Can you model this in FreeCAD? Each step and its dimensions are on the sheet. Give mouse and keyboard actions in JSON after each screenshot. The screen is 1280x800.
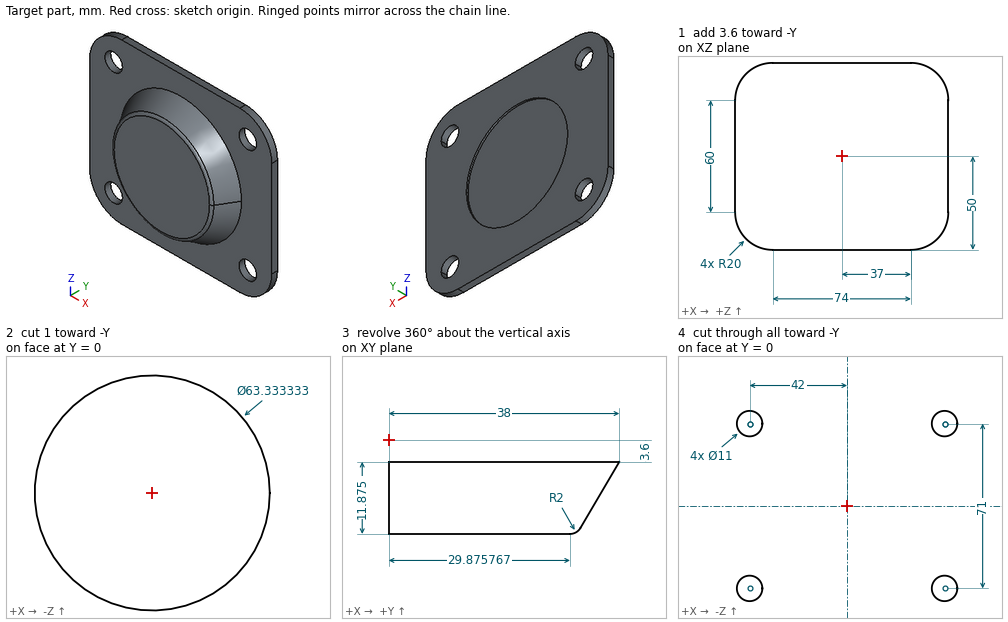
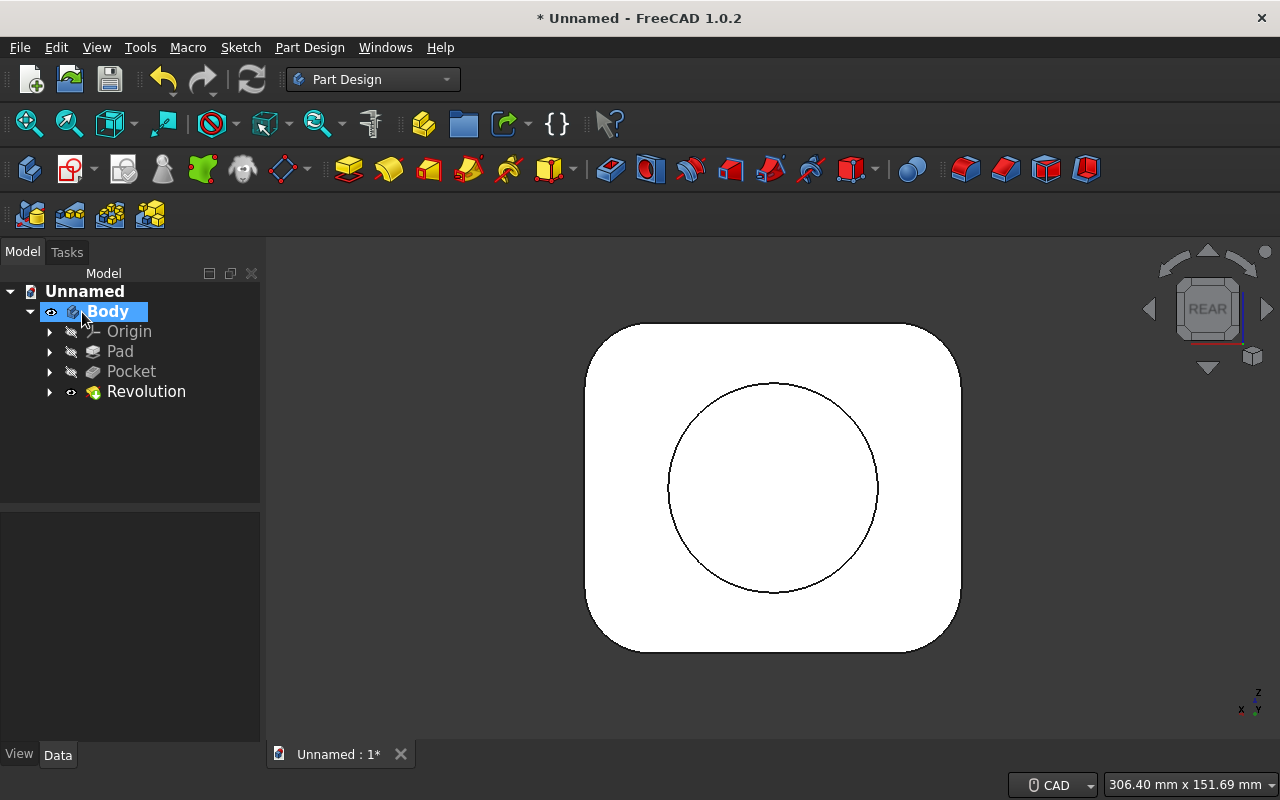
{"action": "left_click", "coordinate": [665, 582]}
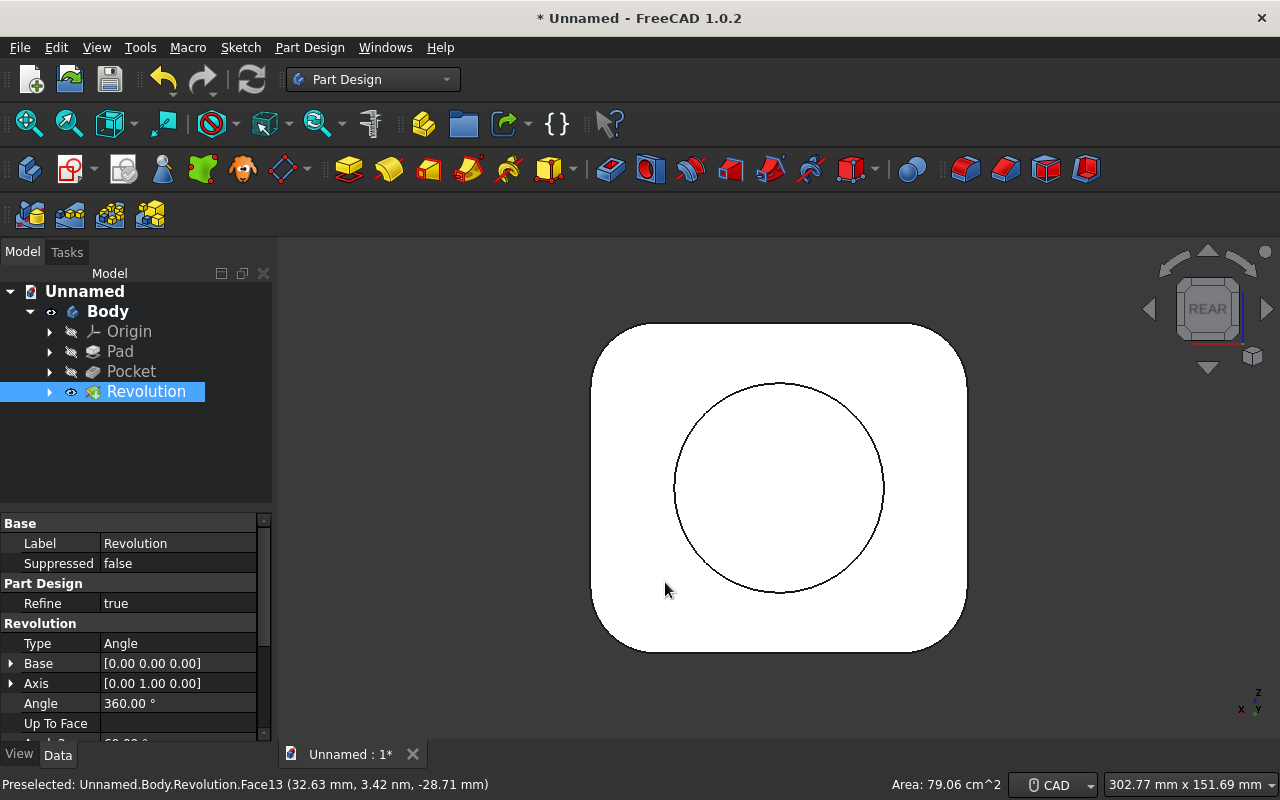
{"action": "left_click", "coordinate": [70, 170]}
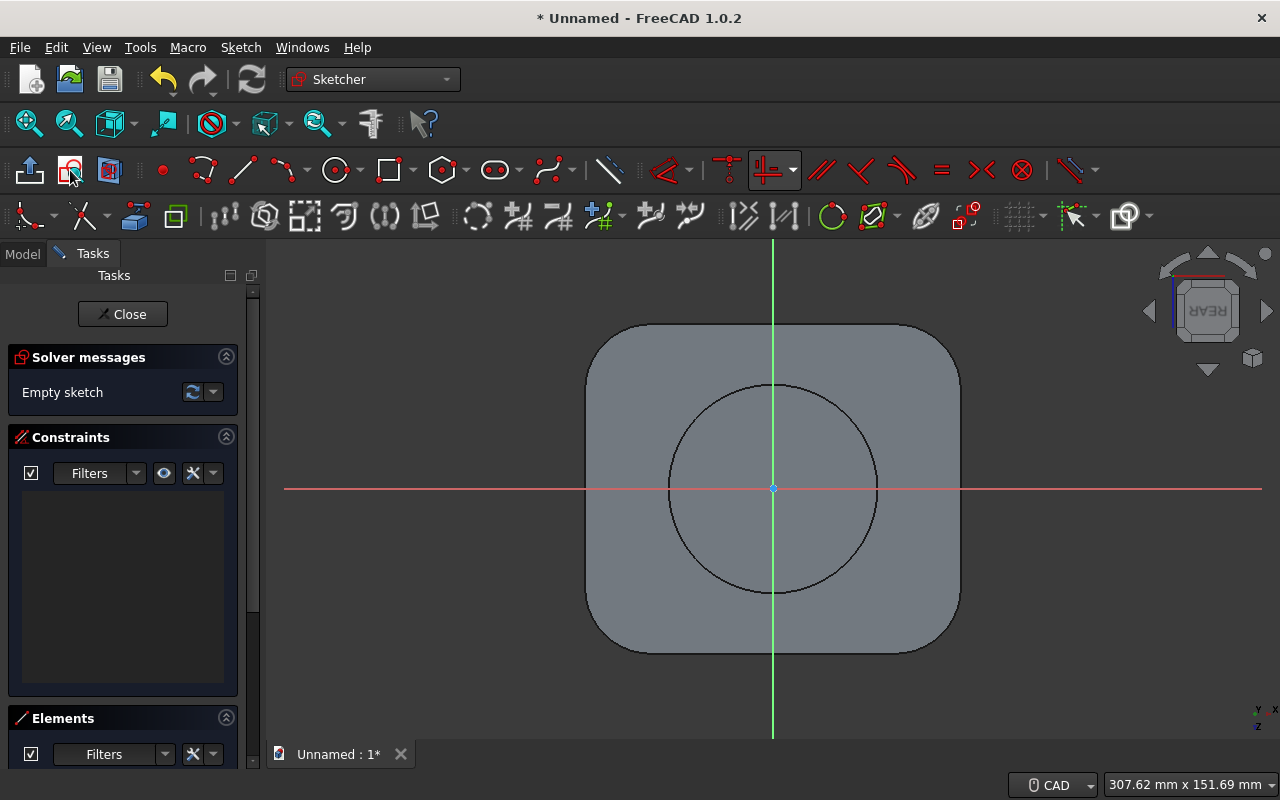
{"action": "left_click", "coordinate": [336, 170]}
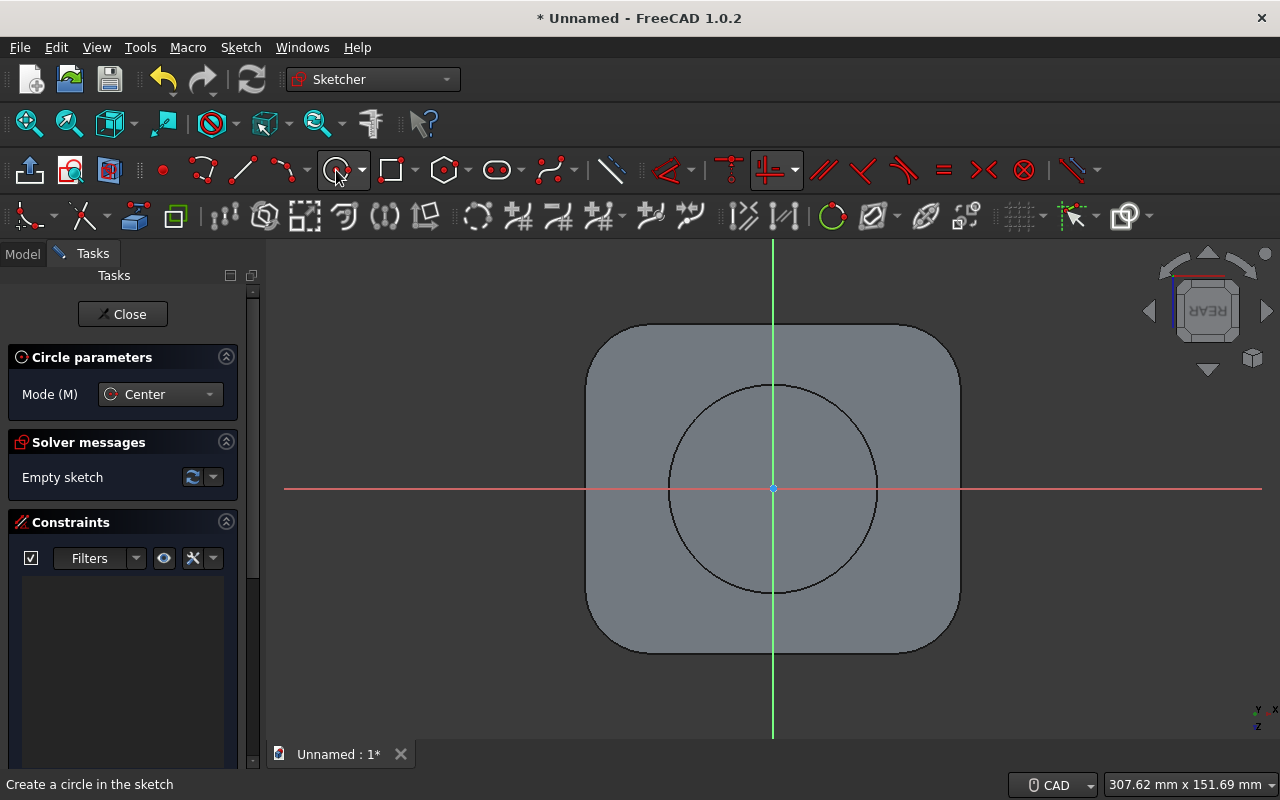
{"action": "scroll", "coordinate": [635, 372], "scroll_direction": "up", "scroll_amount": 2}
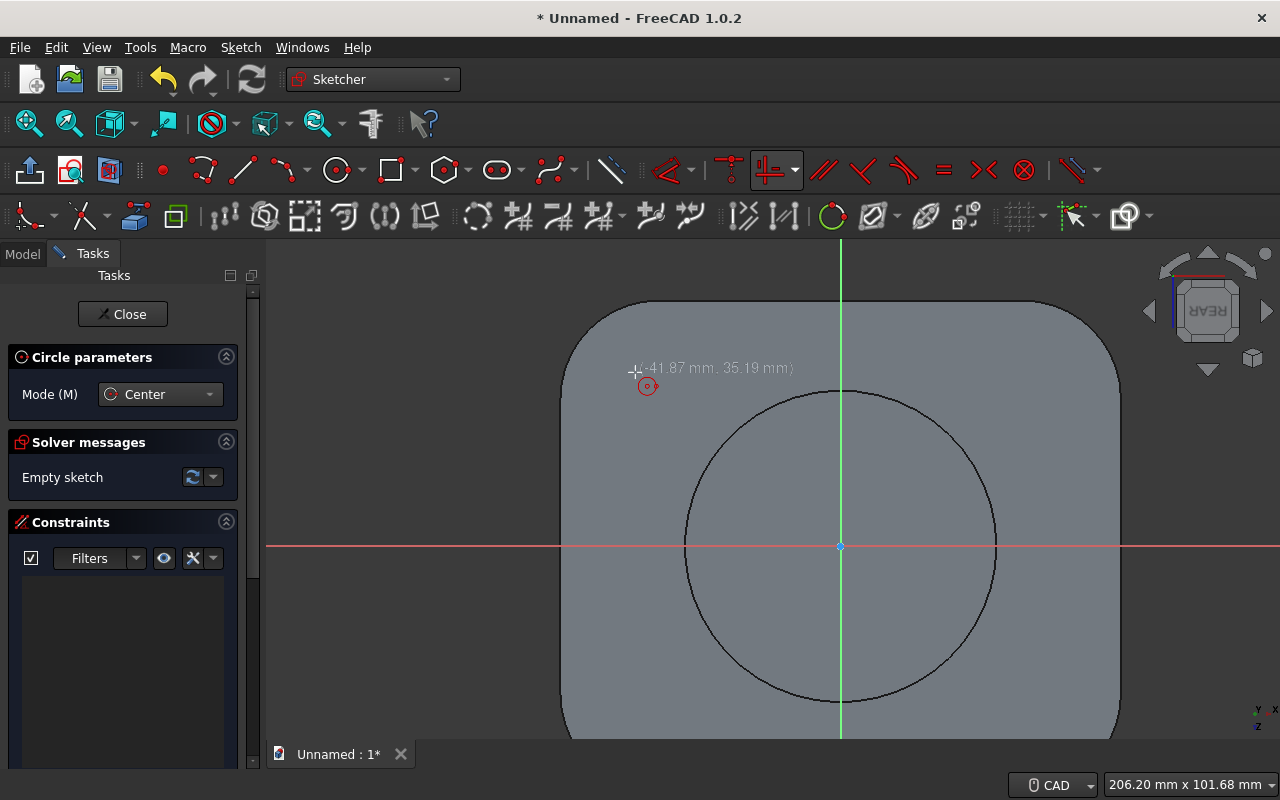
{"action": "left_click", "coordinate": [634, 372]}
{"action": "mouse_move", "coordinate": [653, 353]}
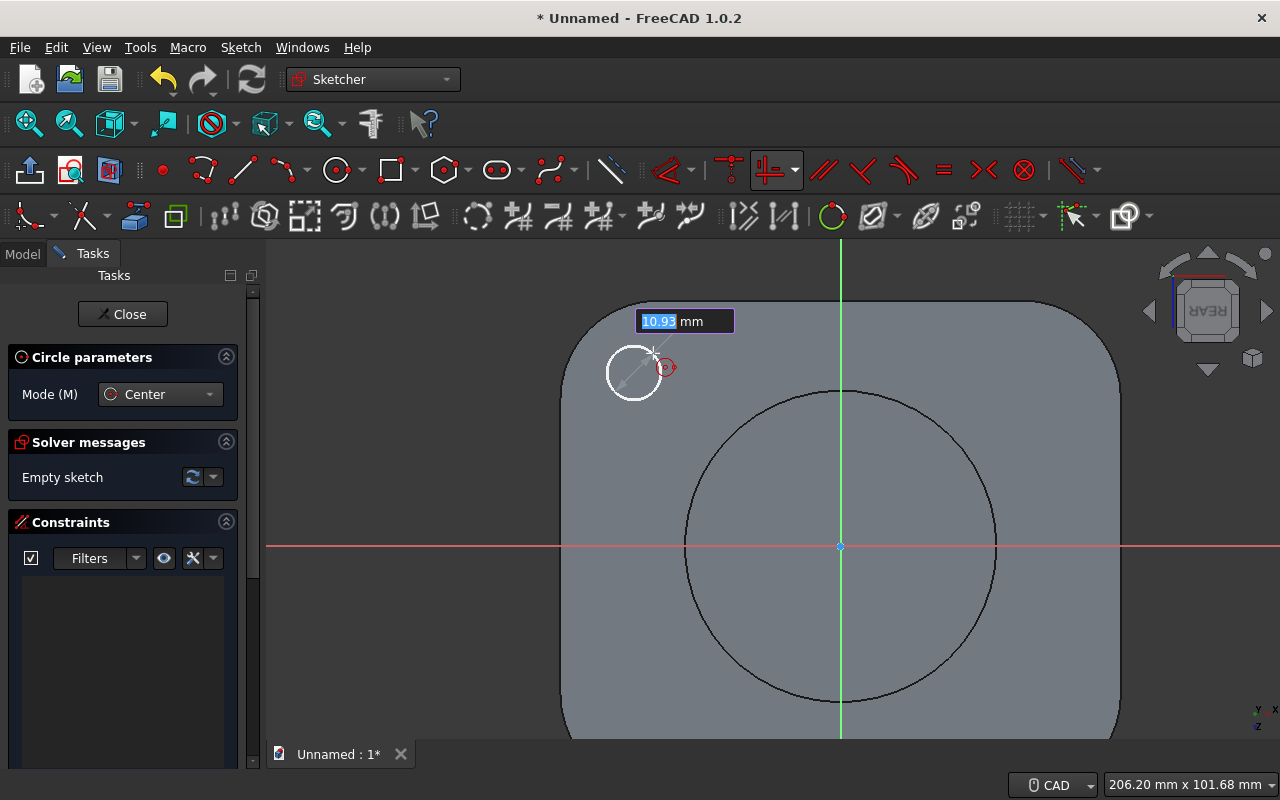
{"action": "type", "text": "11"}
{"action": "key", "text": "Return"}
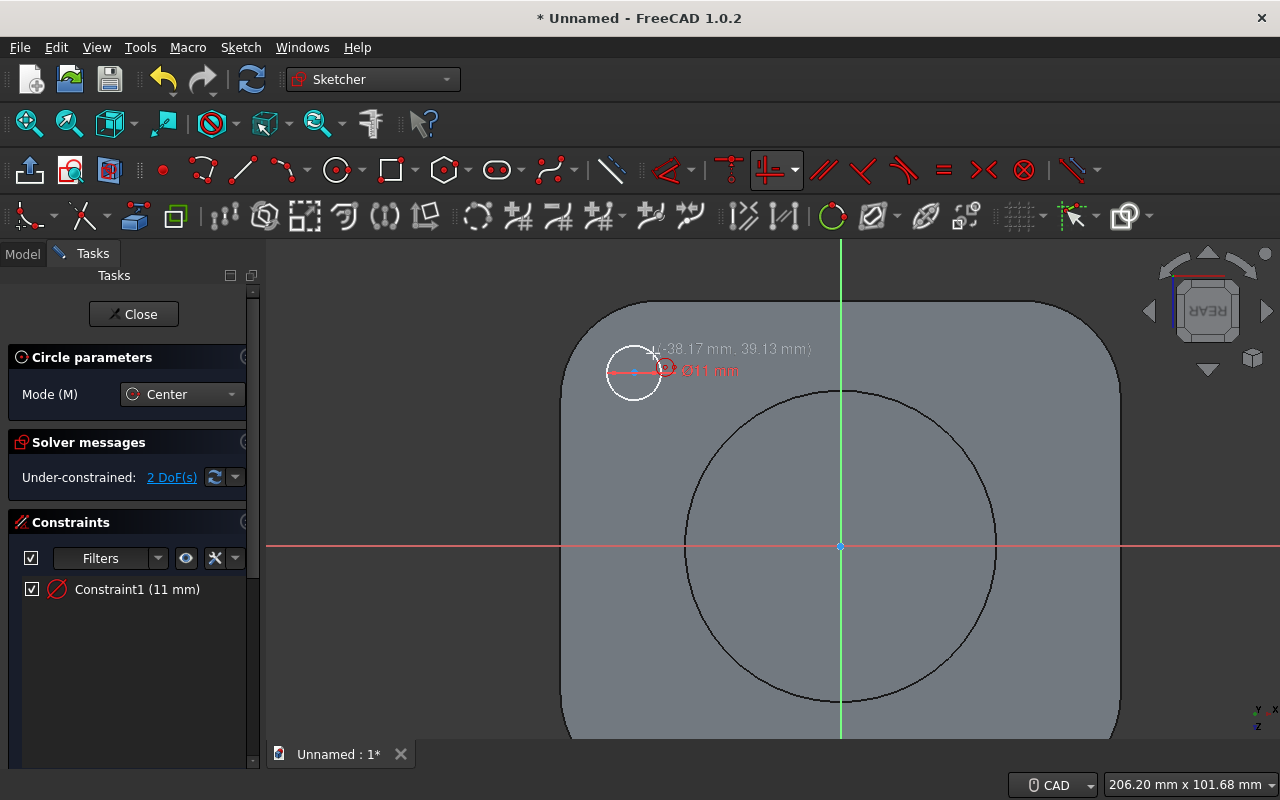
{"action": "left_click", "coordinate": [1047, 372]}
{"action": "mouse_move", "coordinate": [1066, 353]}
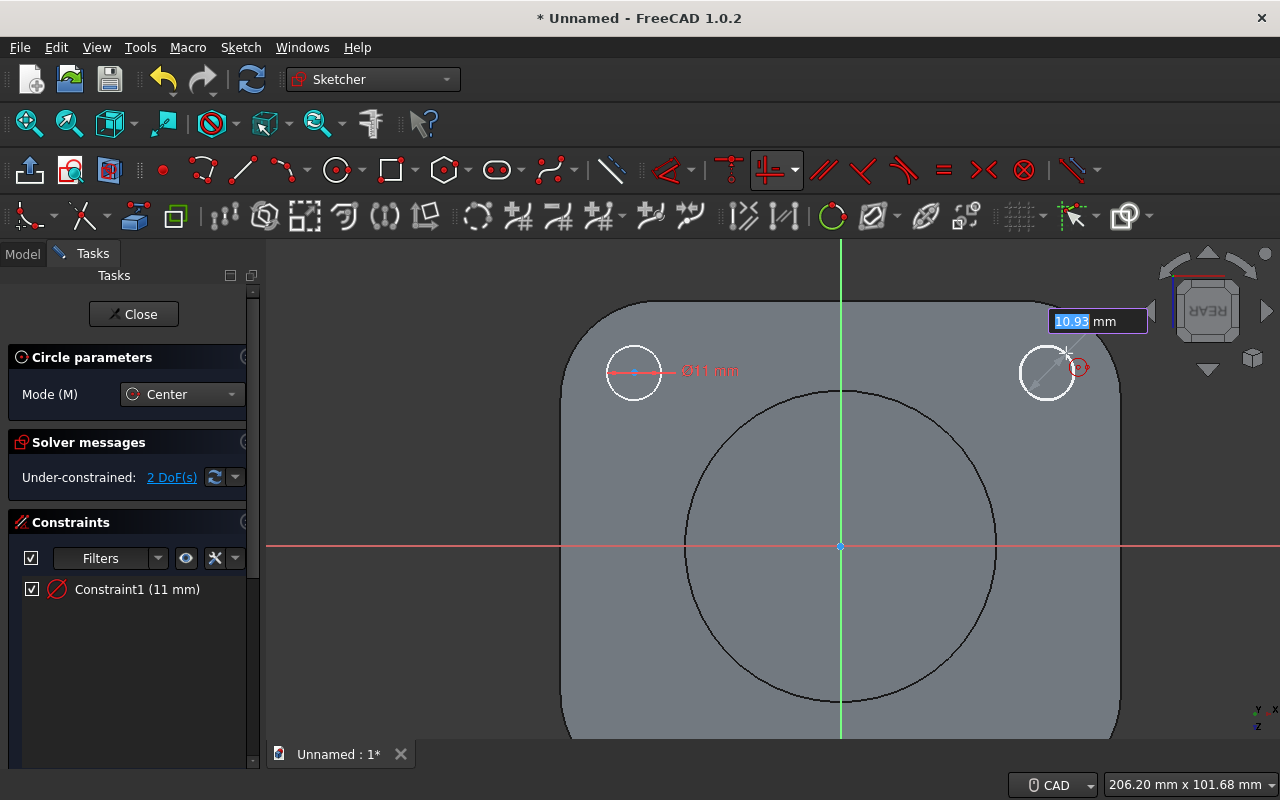
{"action": "type", "text": "11"}
{"action": "key", "text": "Return"}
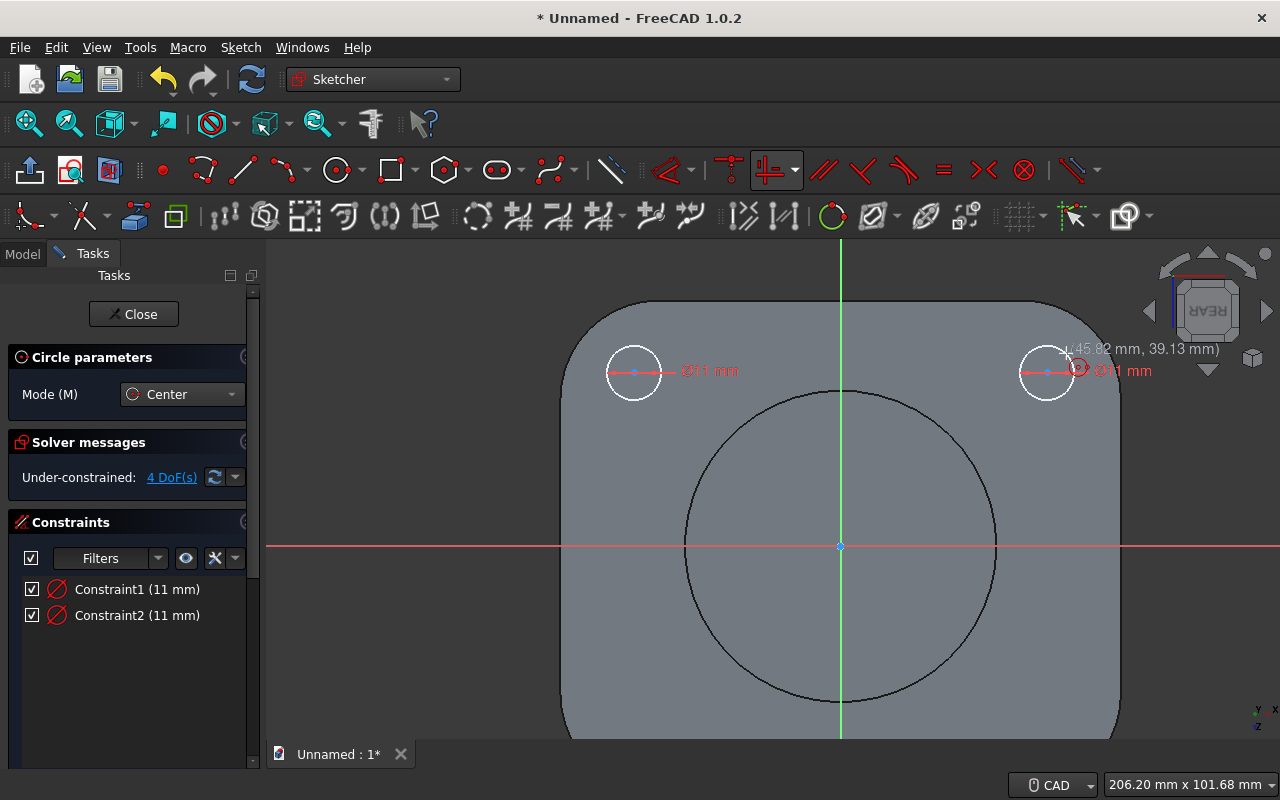
{"action": "scroll", "coordinate": [294, 267], "scroll_direction": "down", "scroll_amount": 1}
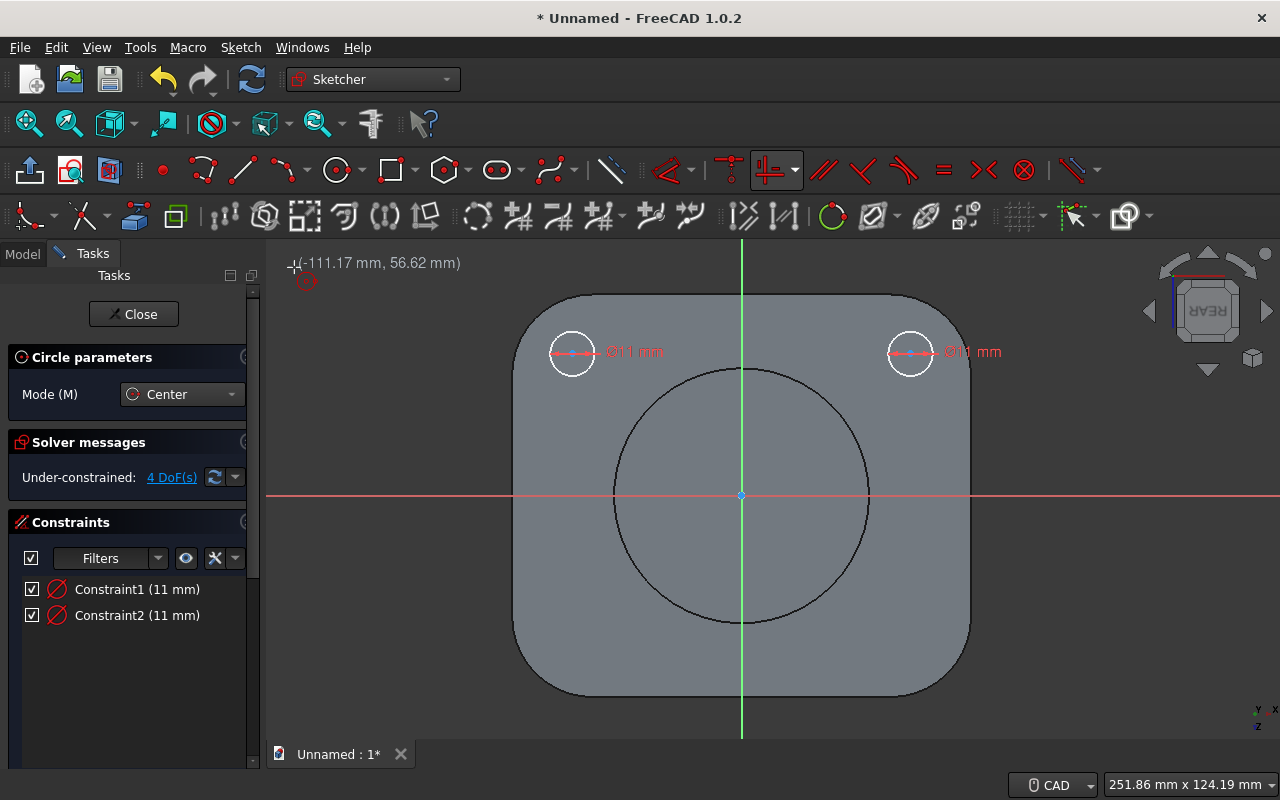
{"action": "left_click", "coordinate": [911, 639]}
{"action": "mouse_move", "coordinate": [926, 623]}